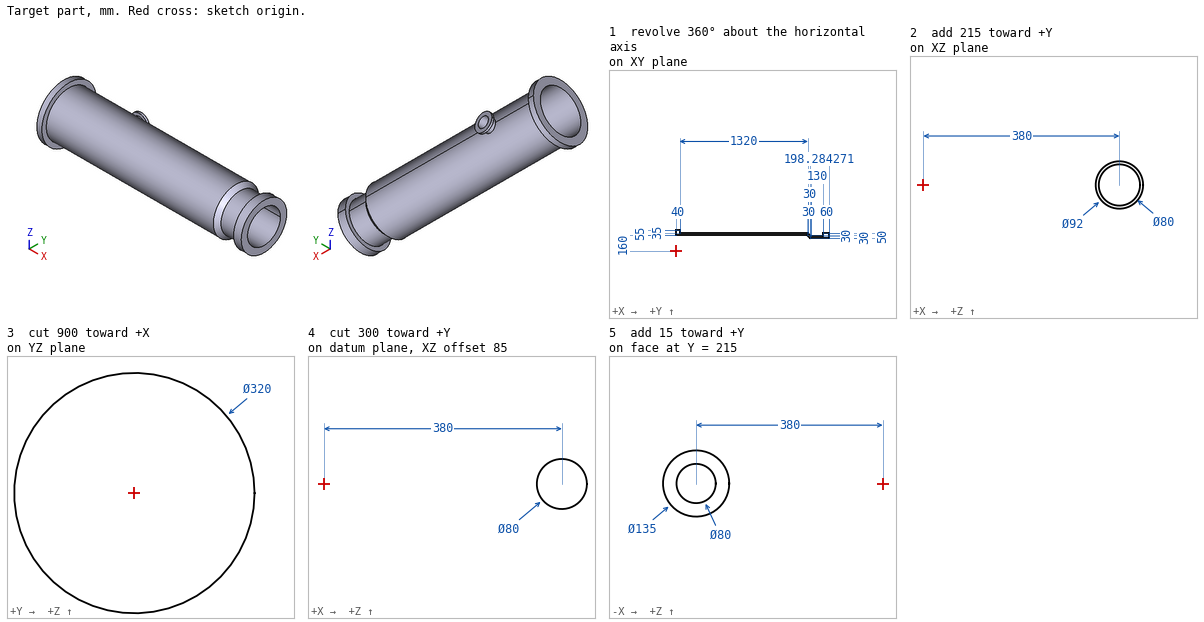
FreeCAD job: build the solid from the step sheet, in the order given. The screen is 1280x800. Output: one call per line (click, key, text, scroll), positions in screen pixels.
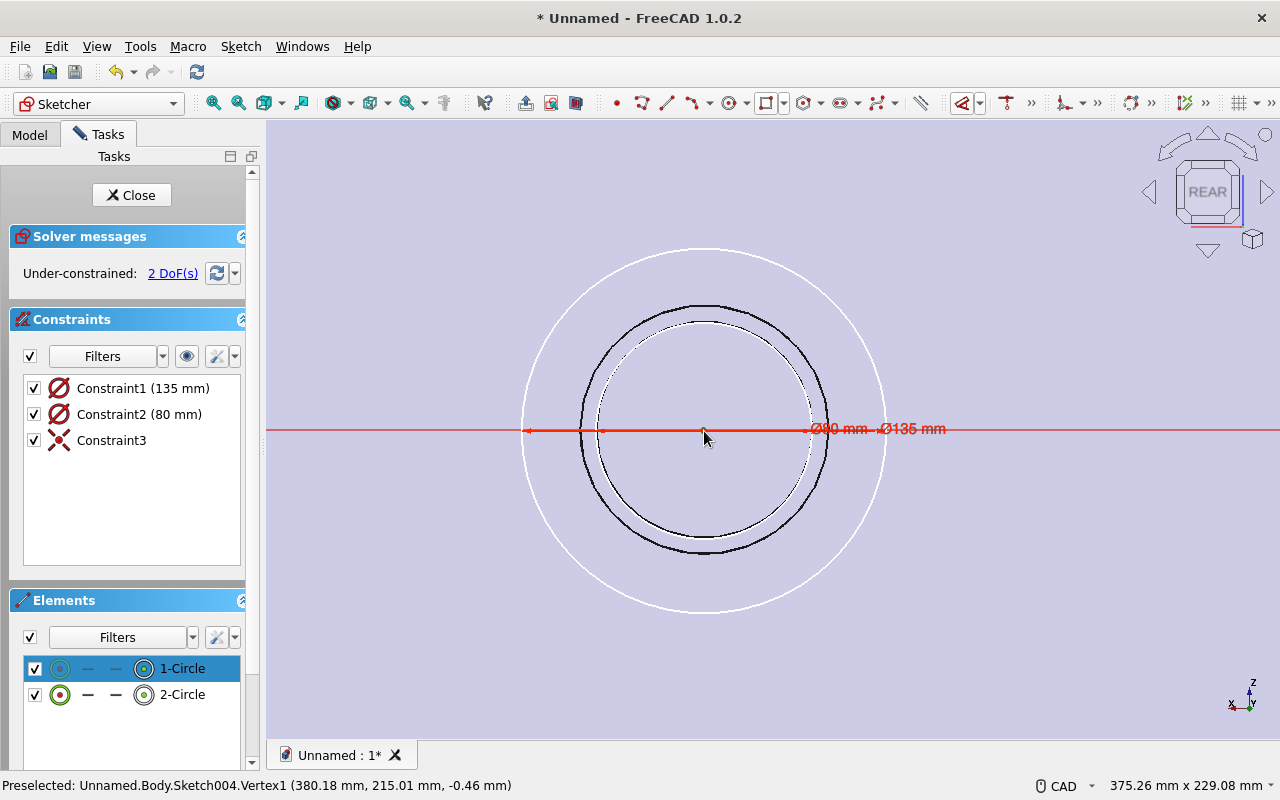
click(353, 430)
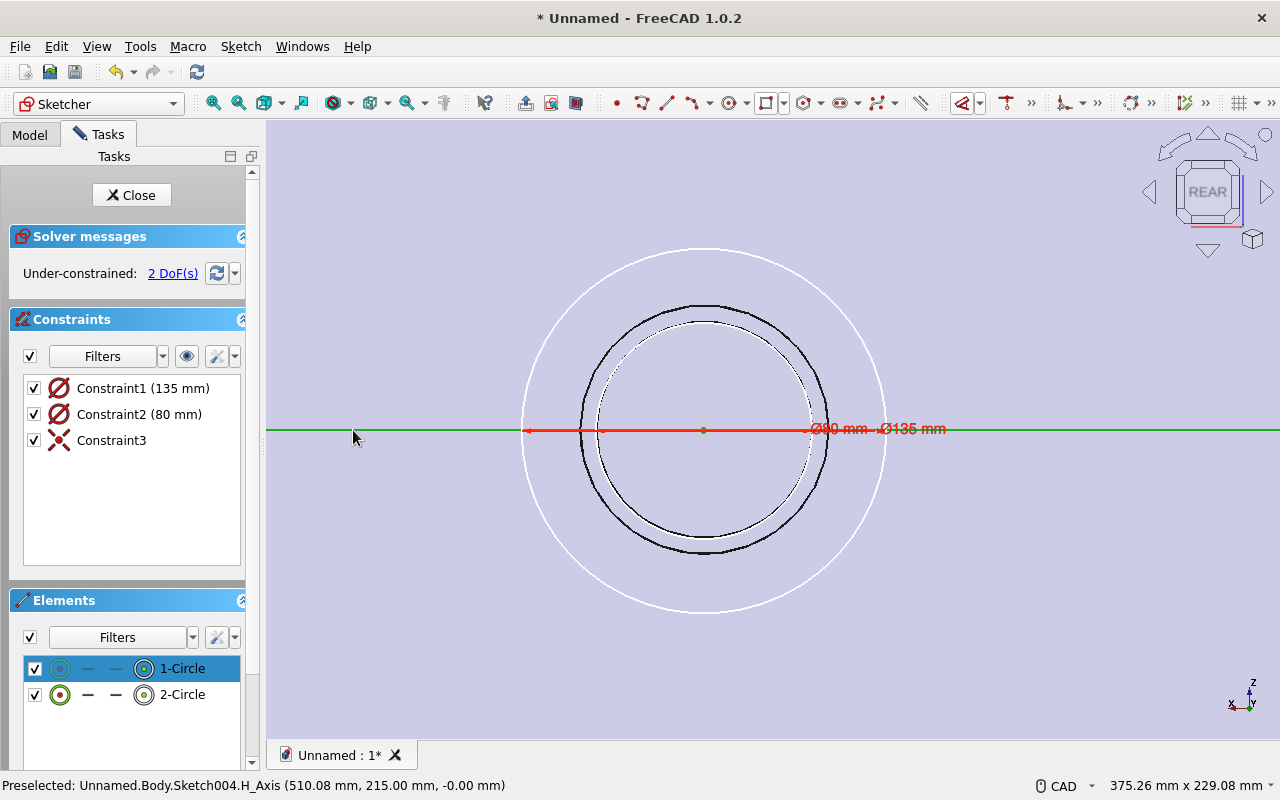
key(c)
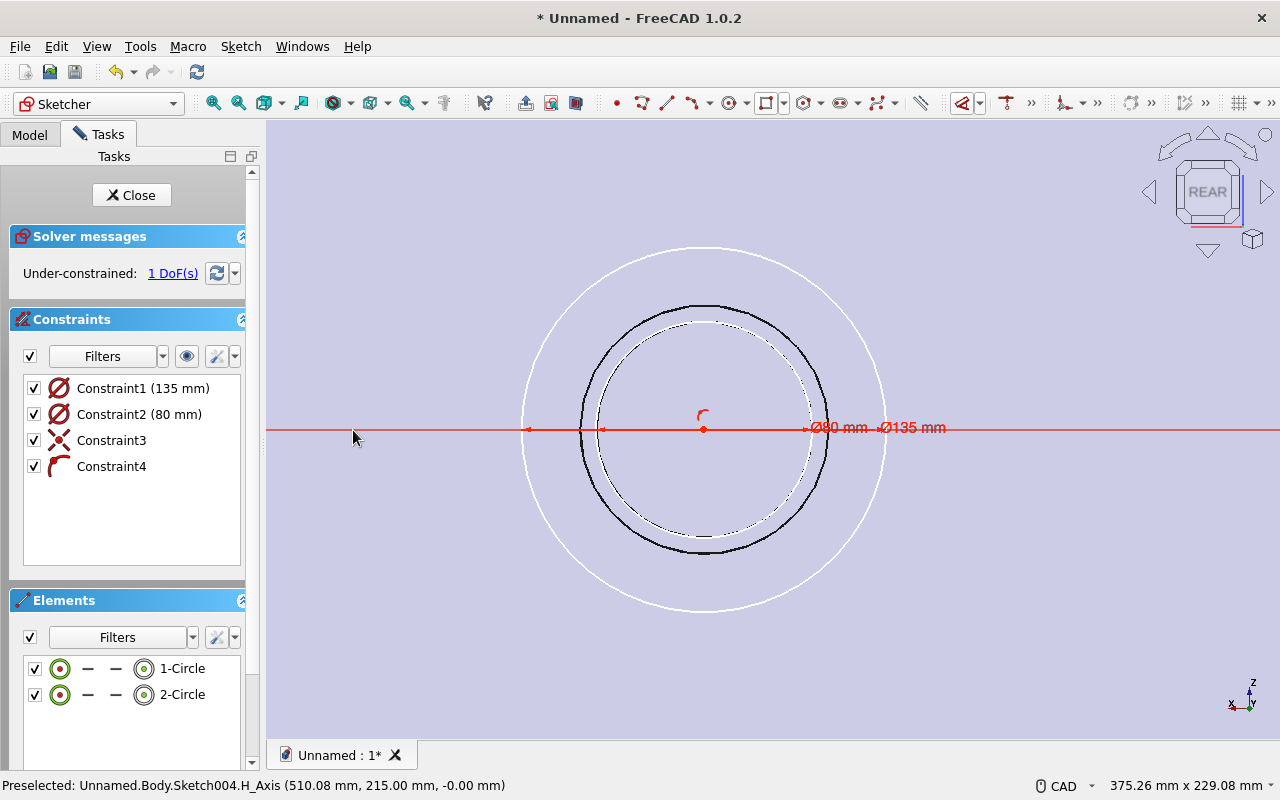
click(704, 430)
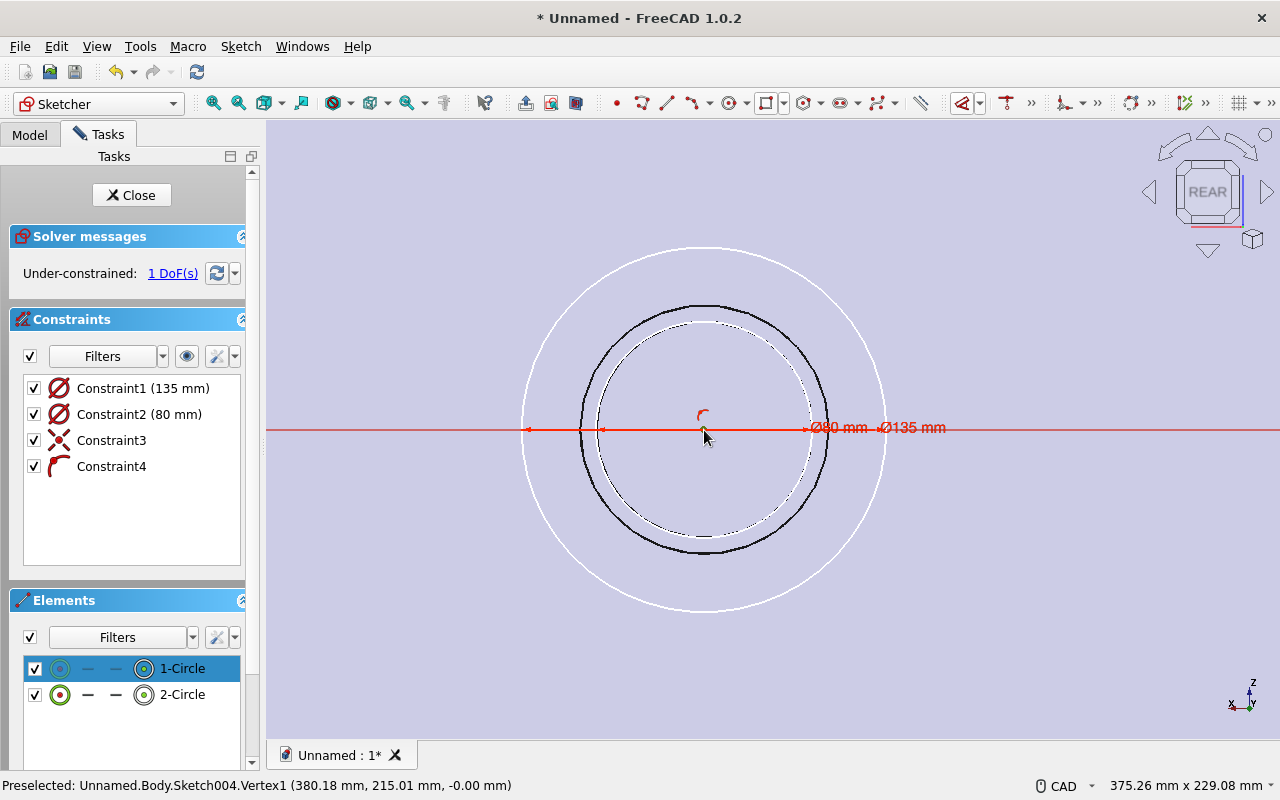
key(l)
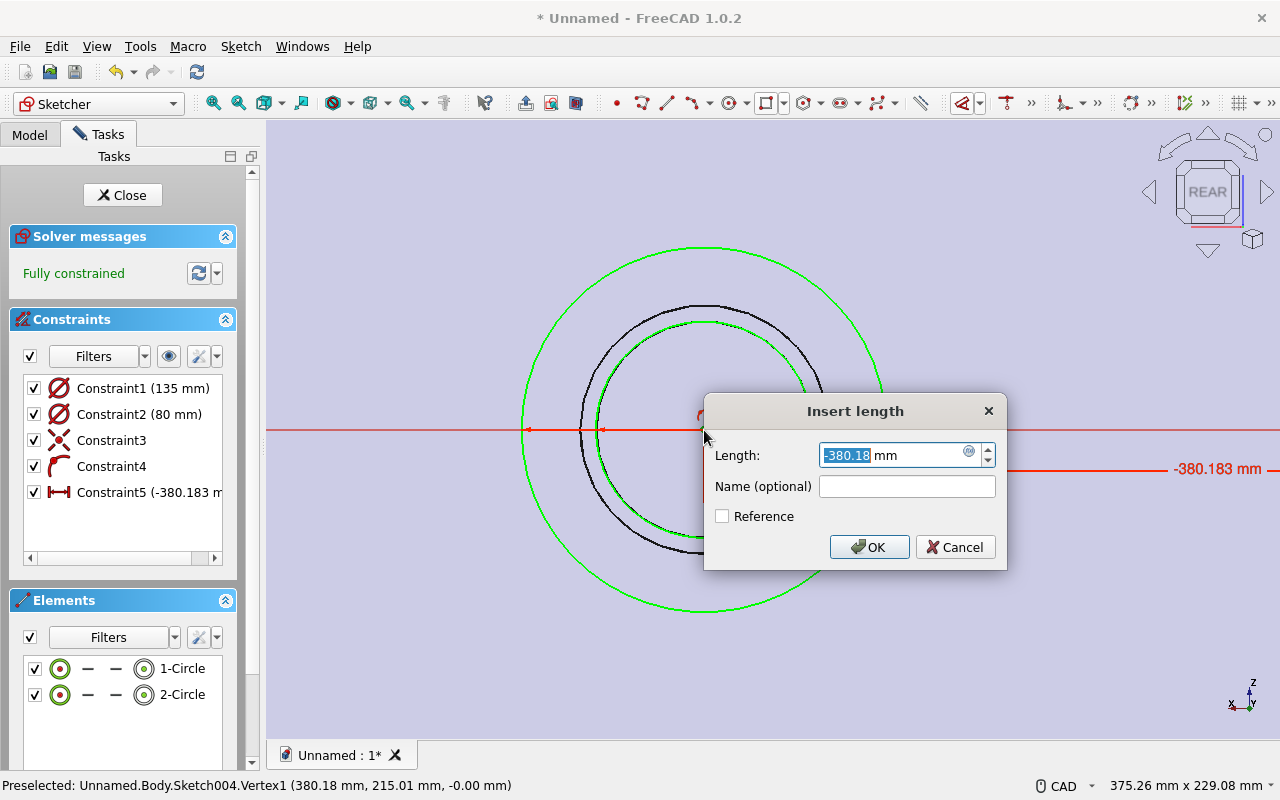
text(-380)
key(Return)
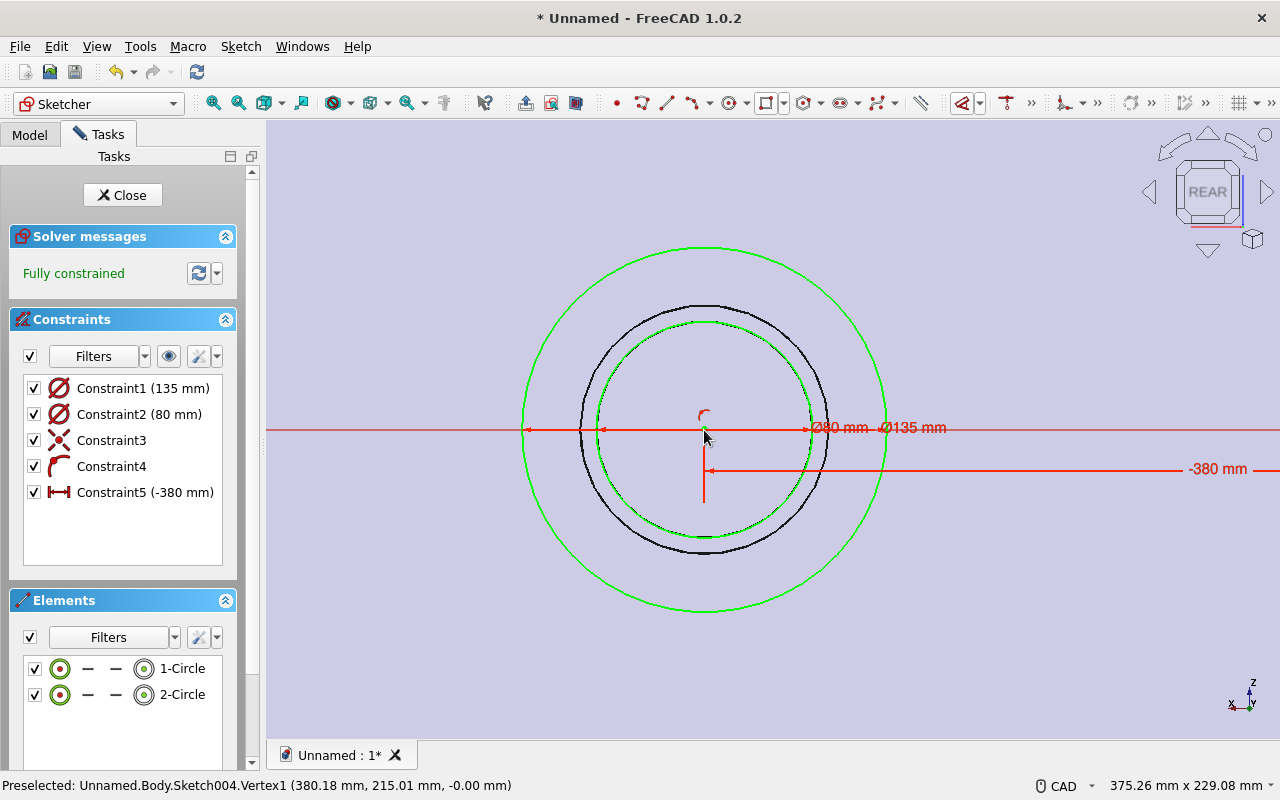
click(123, 195)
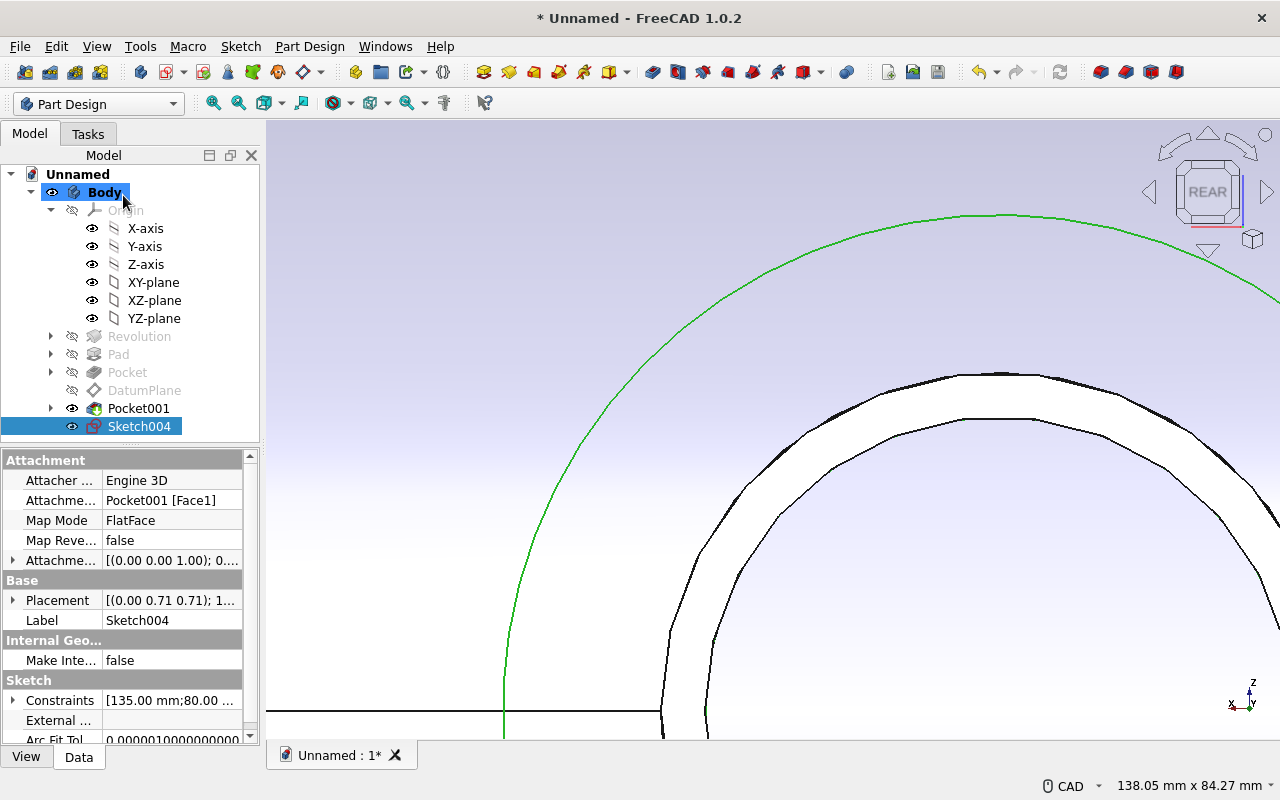
click(484, 72)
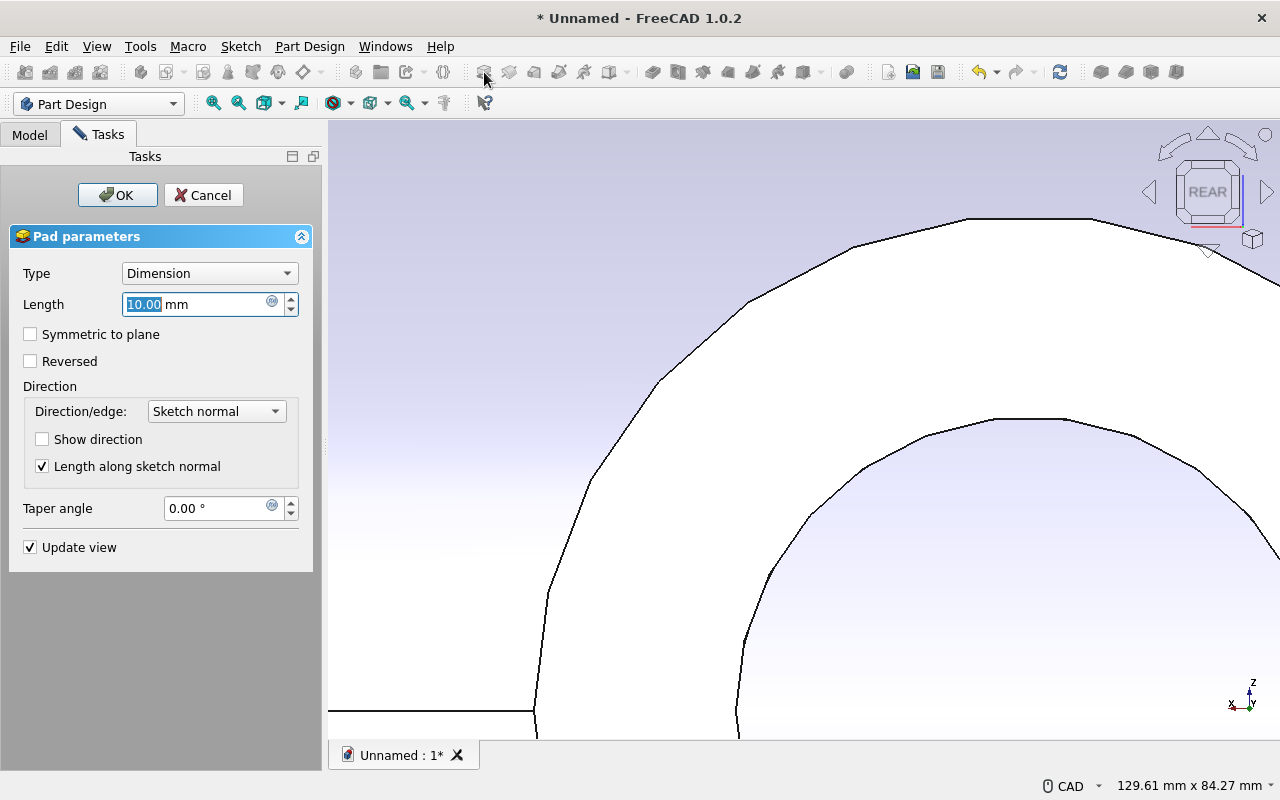
text(15)
key(Tab)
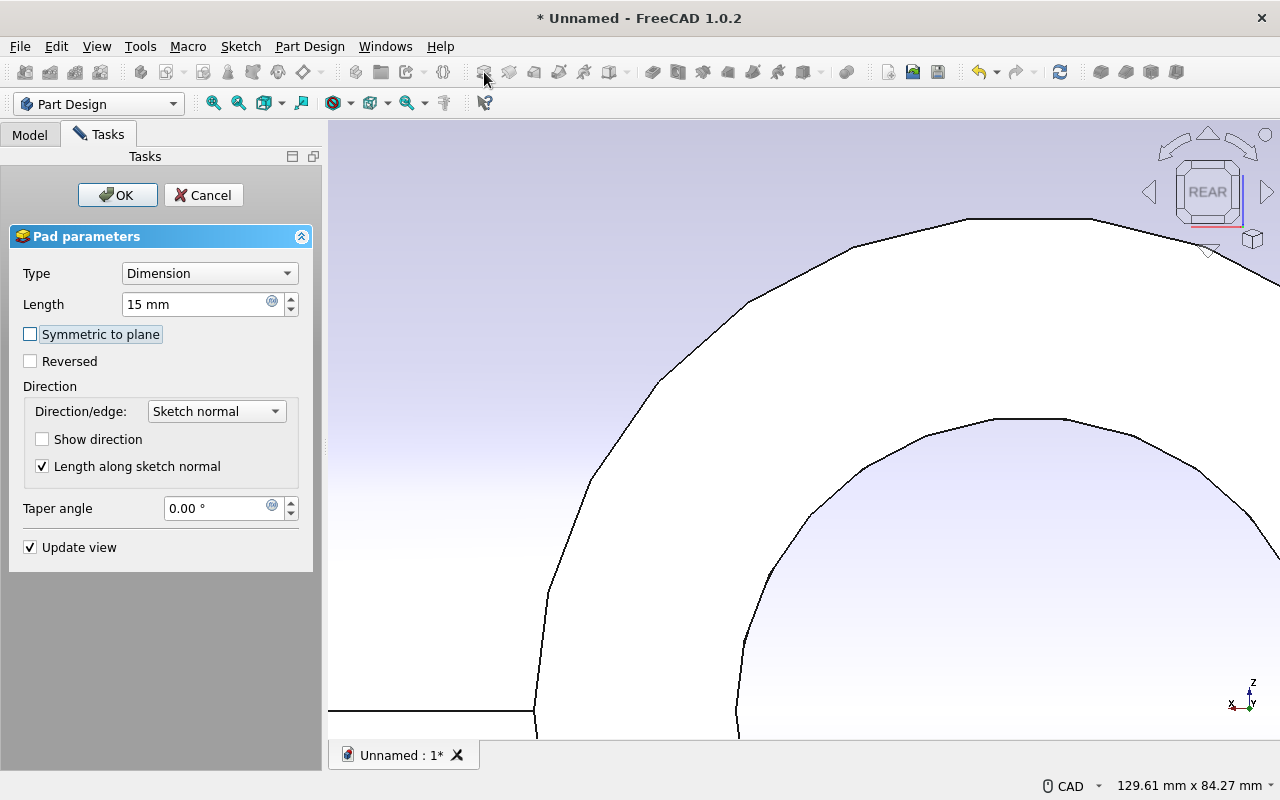
click(118, 195)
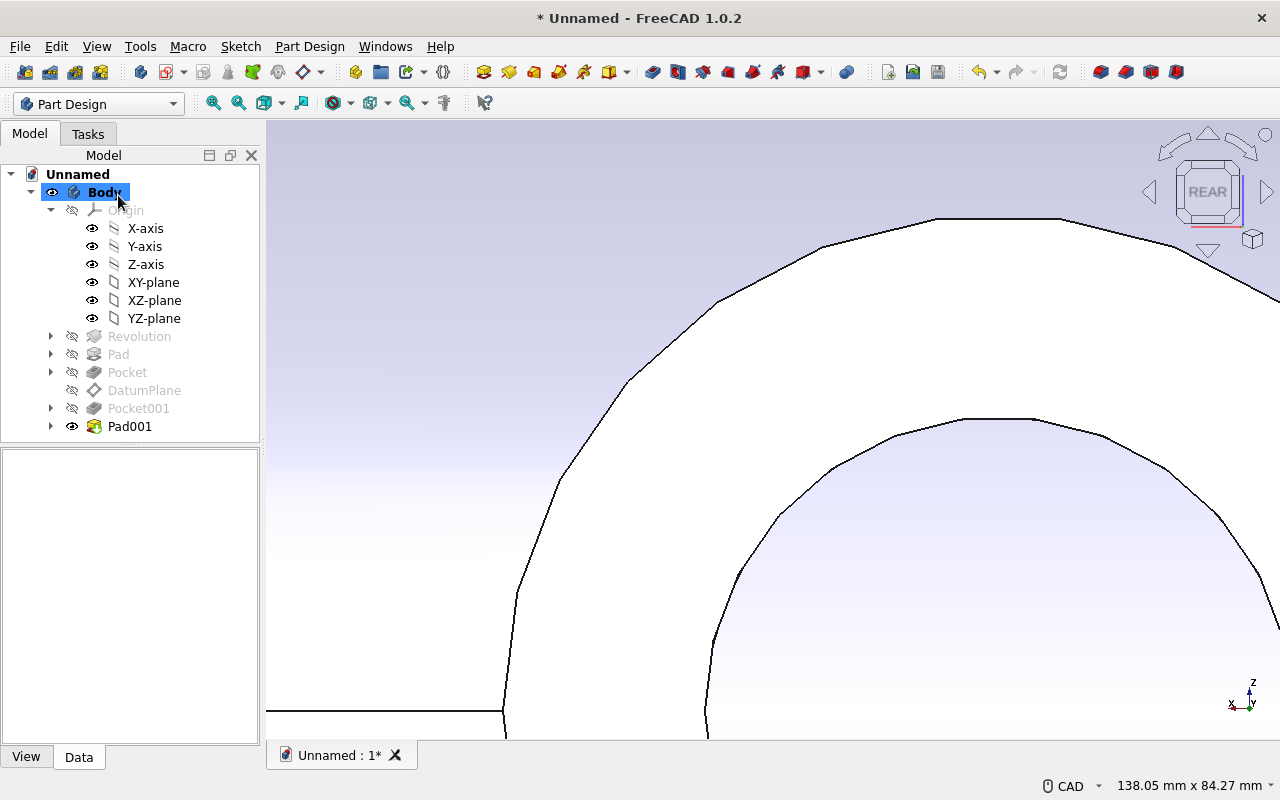
key(0)